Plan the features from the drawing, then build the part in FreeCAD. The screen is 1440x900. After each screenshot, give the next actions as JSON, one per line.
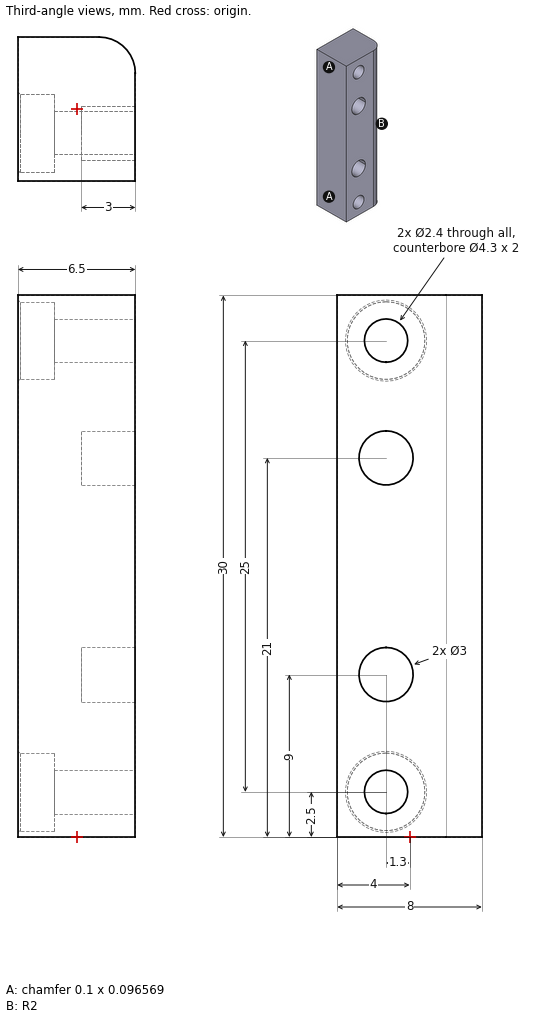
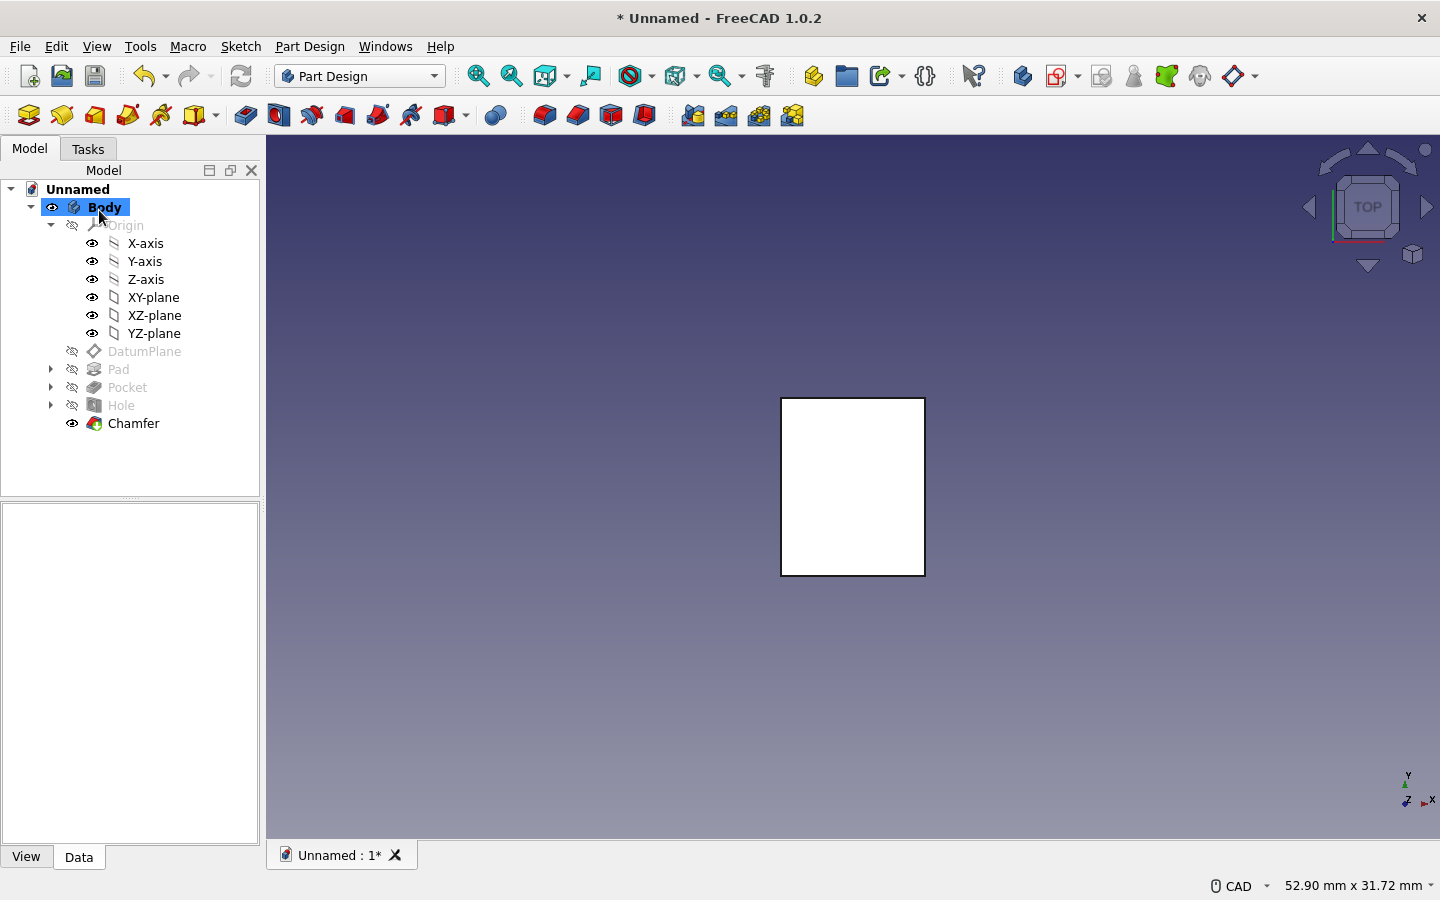
{"action": "left_click", "coordinate": [479, 76]}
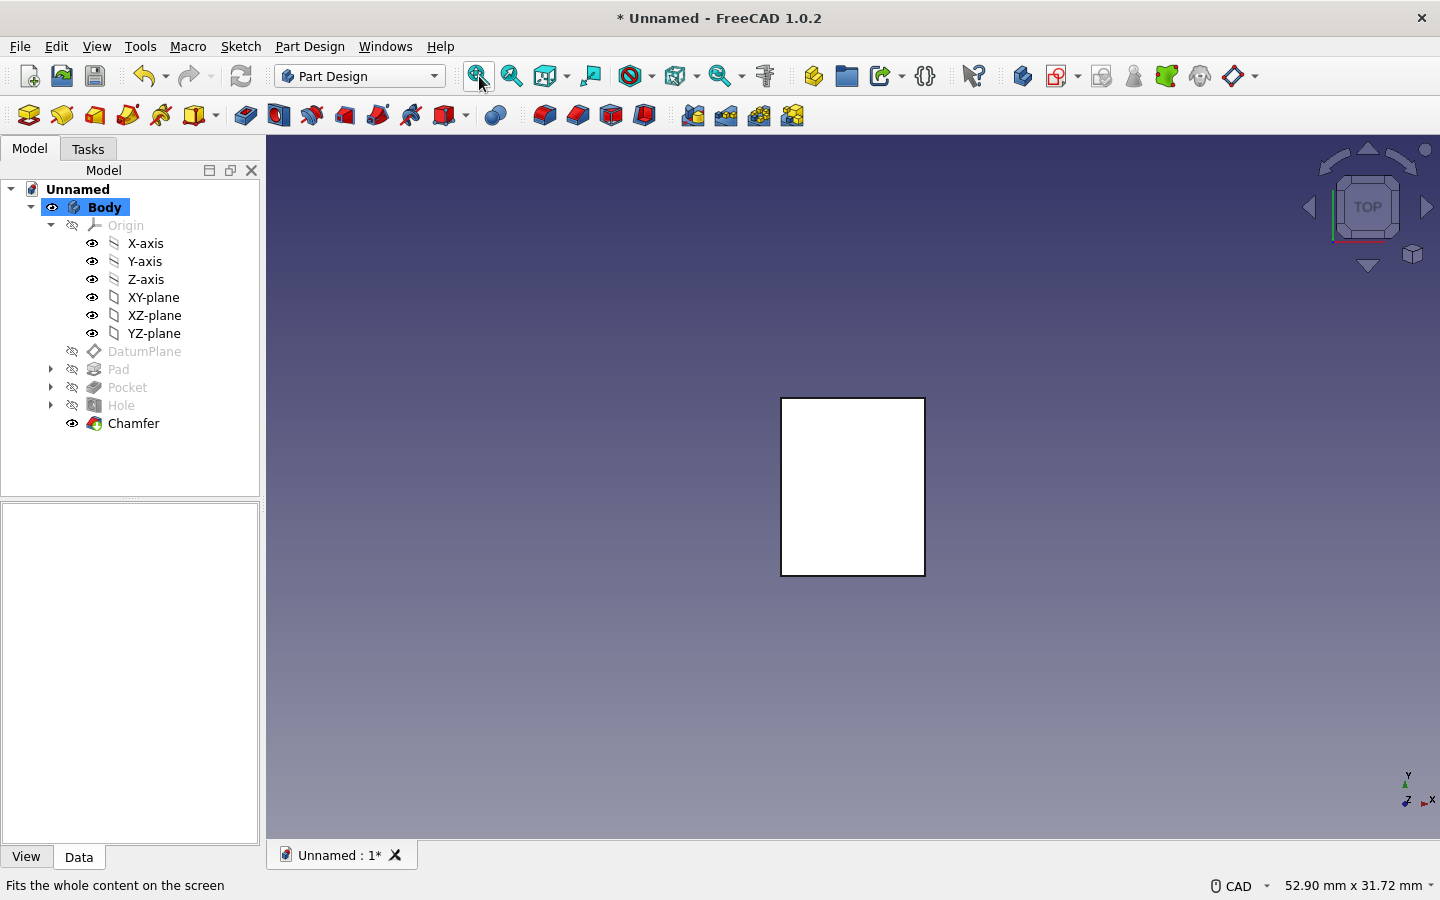
{"action": "key", "text": "1"}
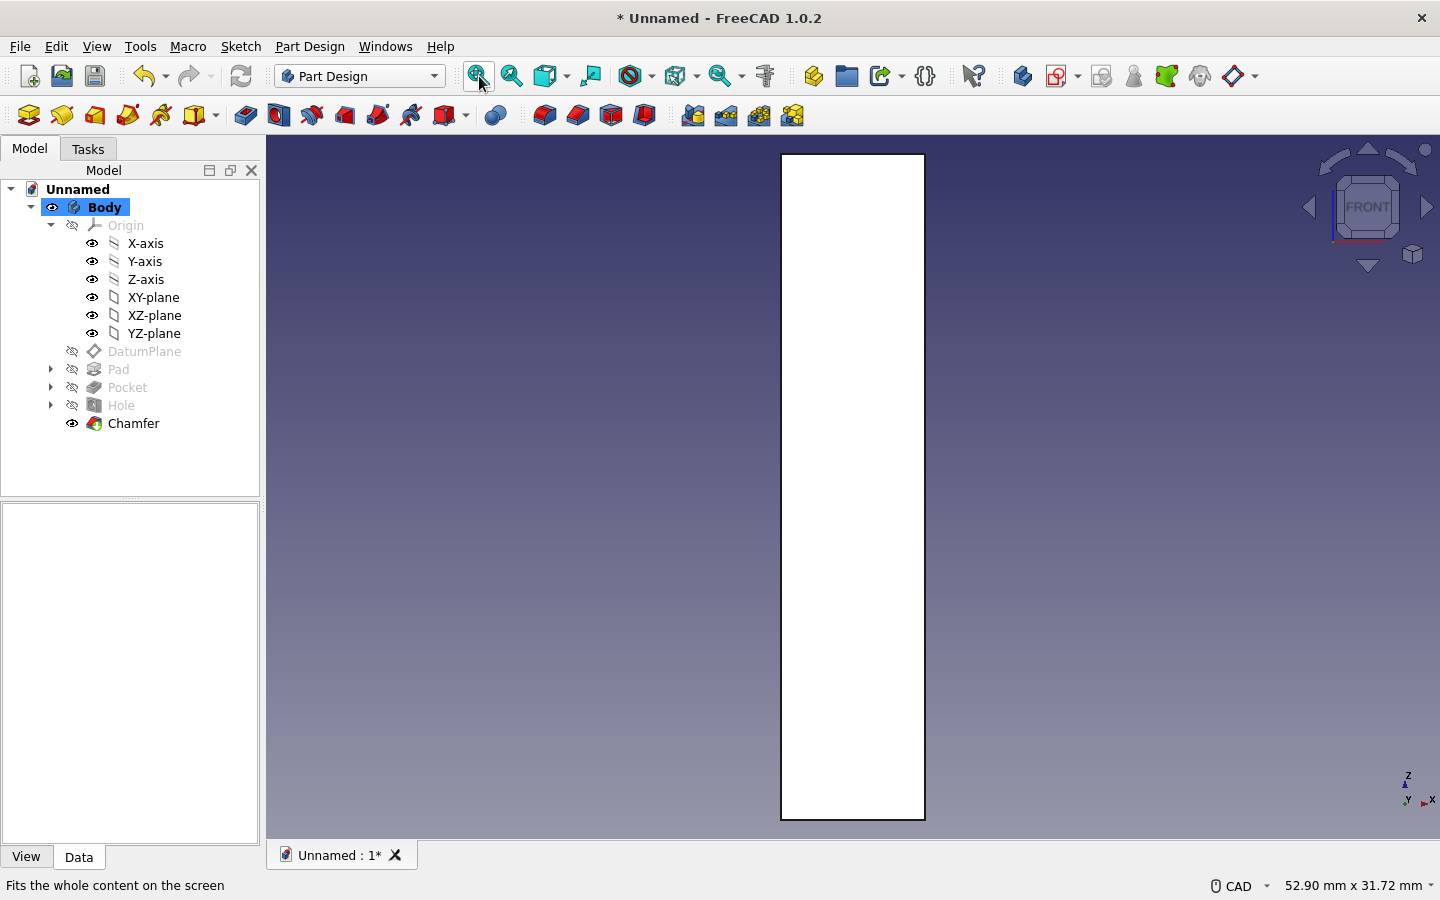
{"action": "key", "text": "3"}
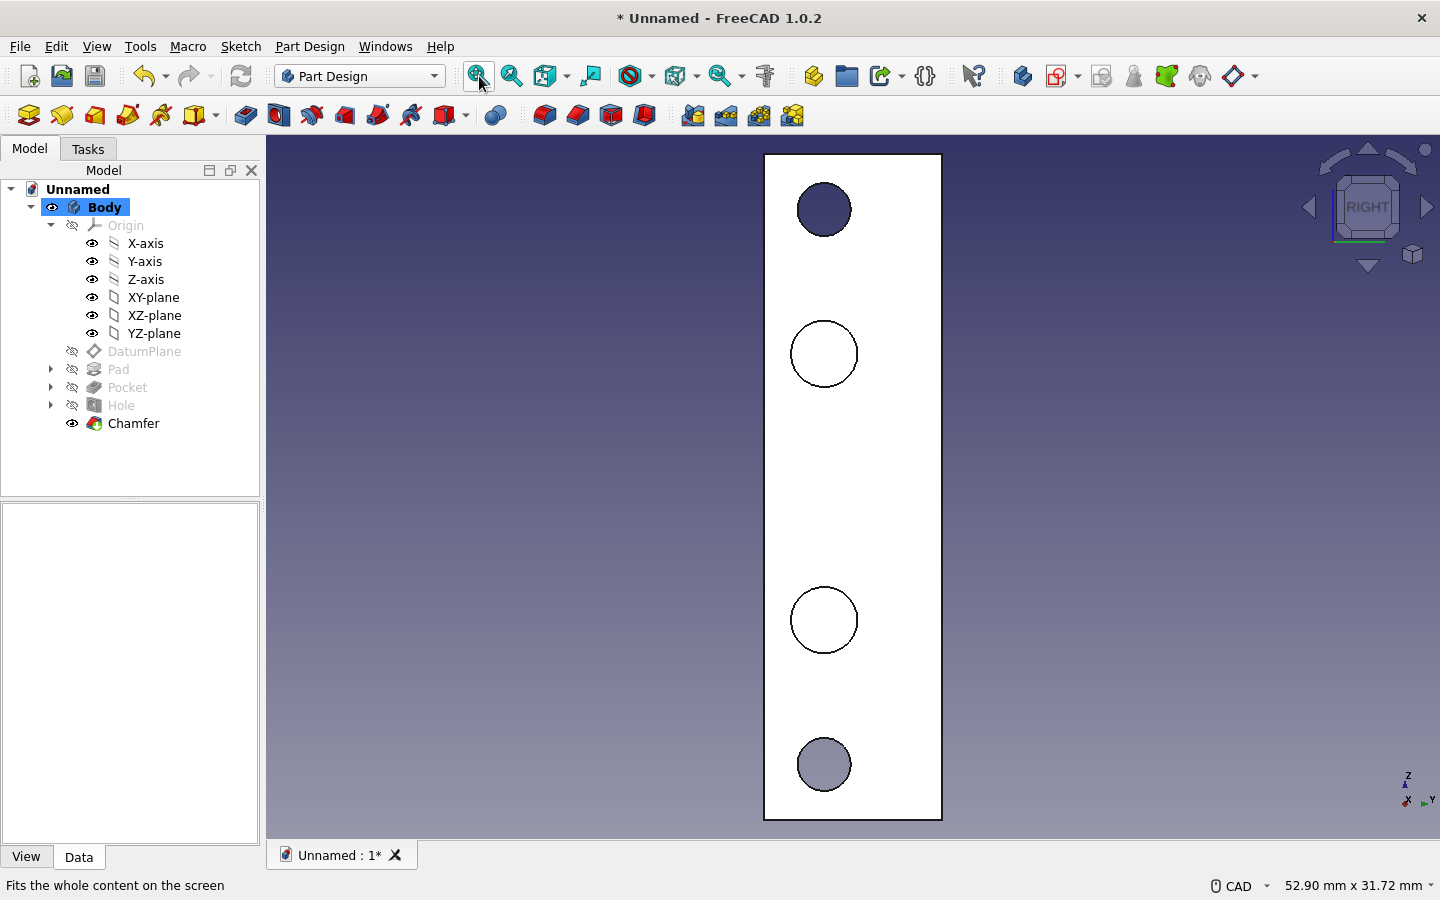
{"action": "key", "text": "5"}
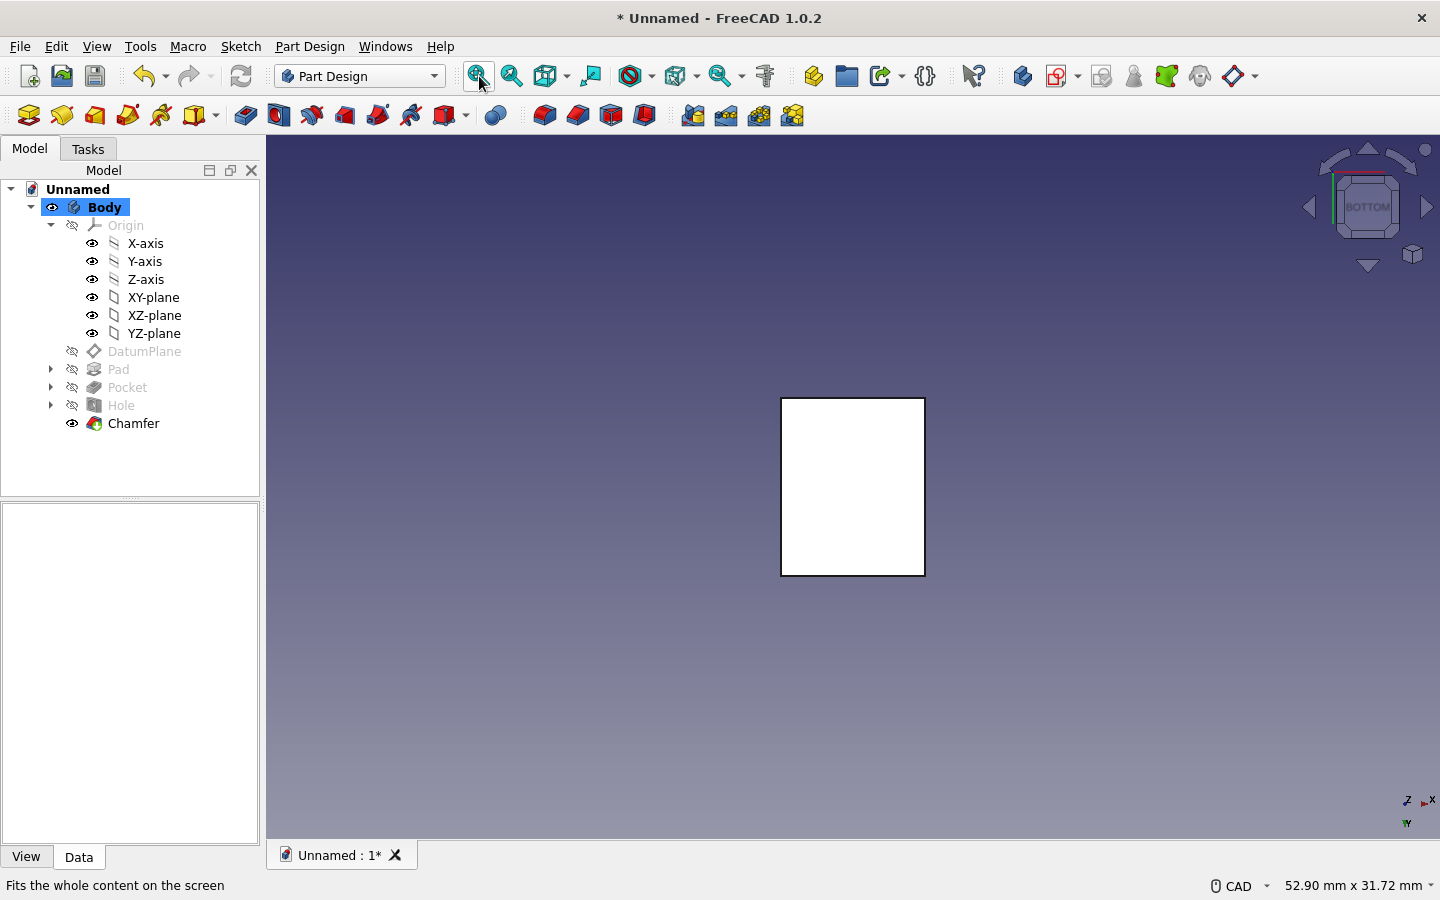
{"action": "left_click", "coordinate": [479, 76]}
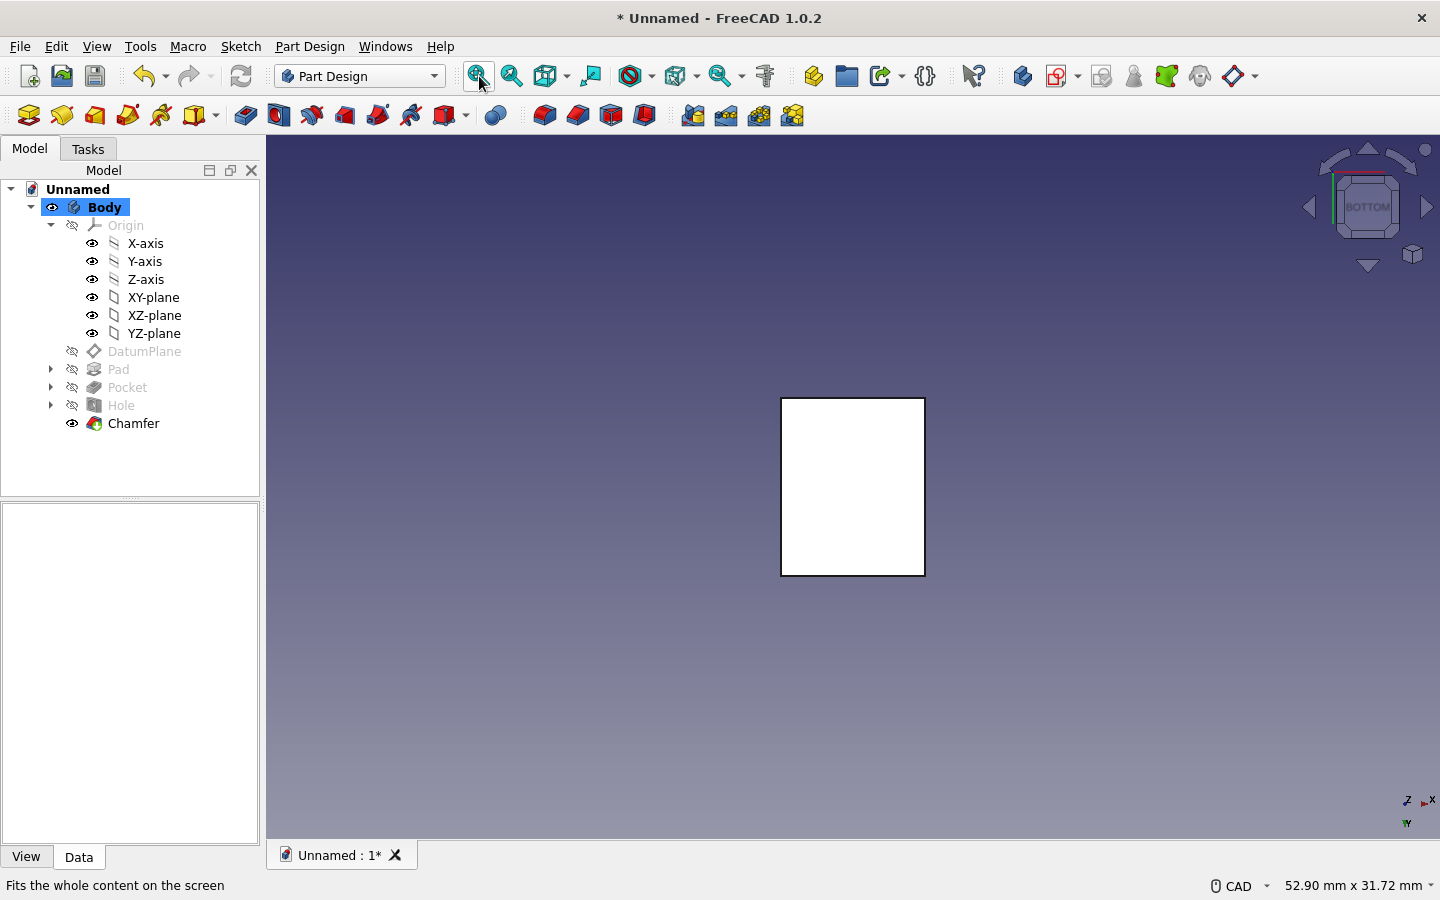
{"action": "key", "text": "4"}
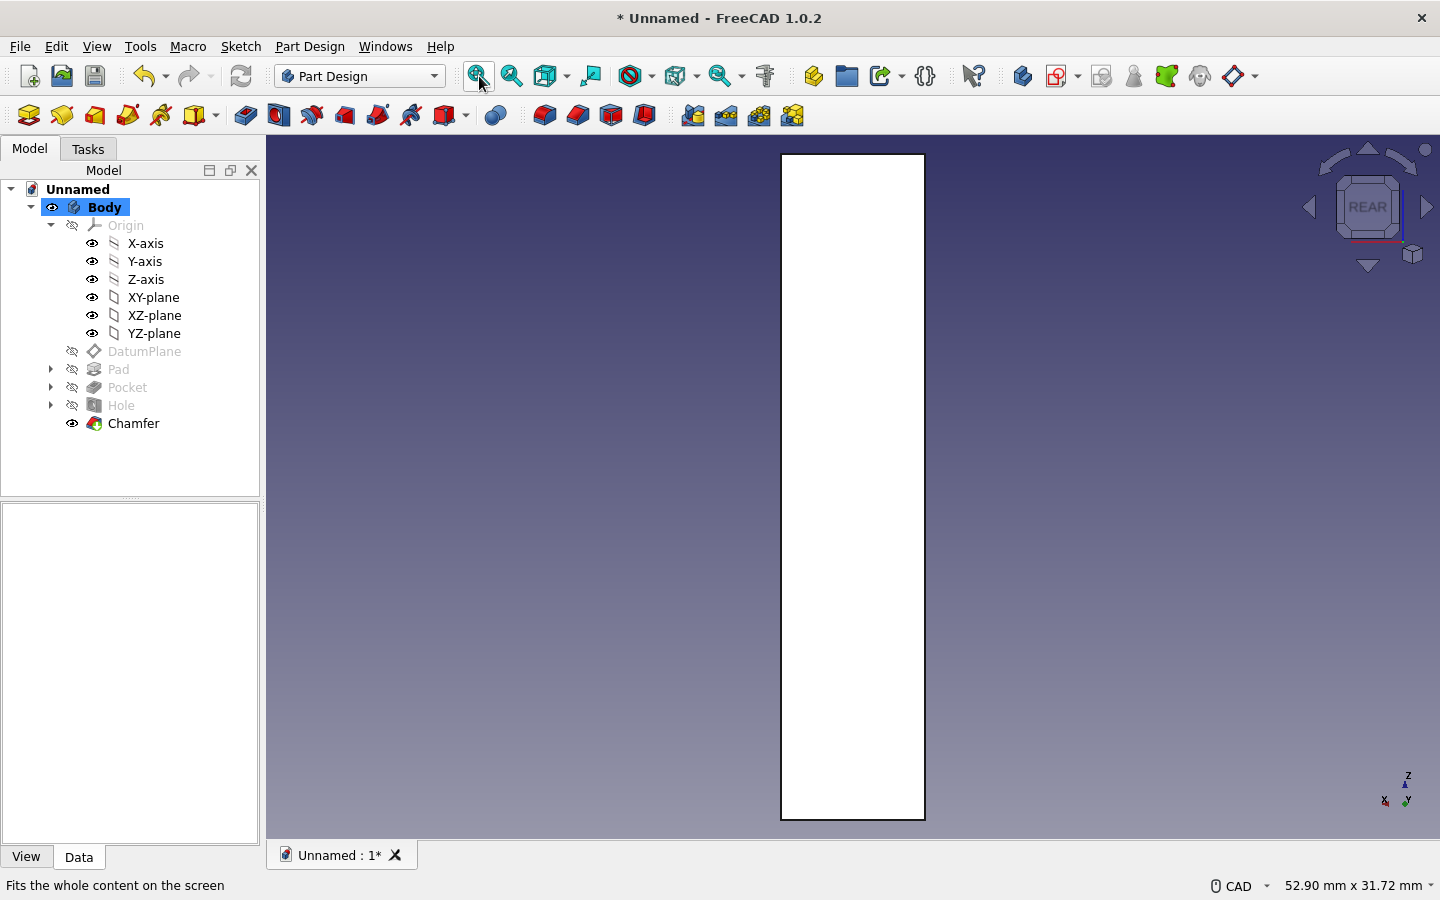
{"action": "left_click", "coordinate": [781, 486]}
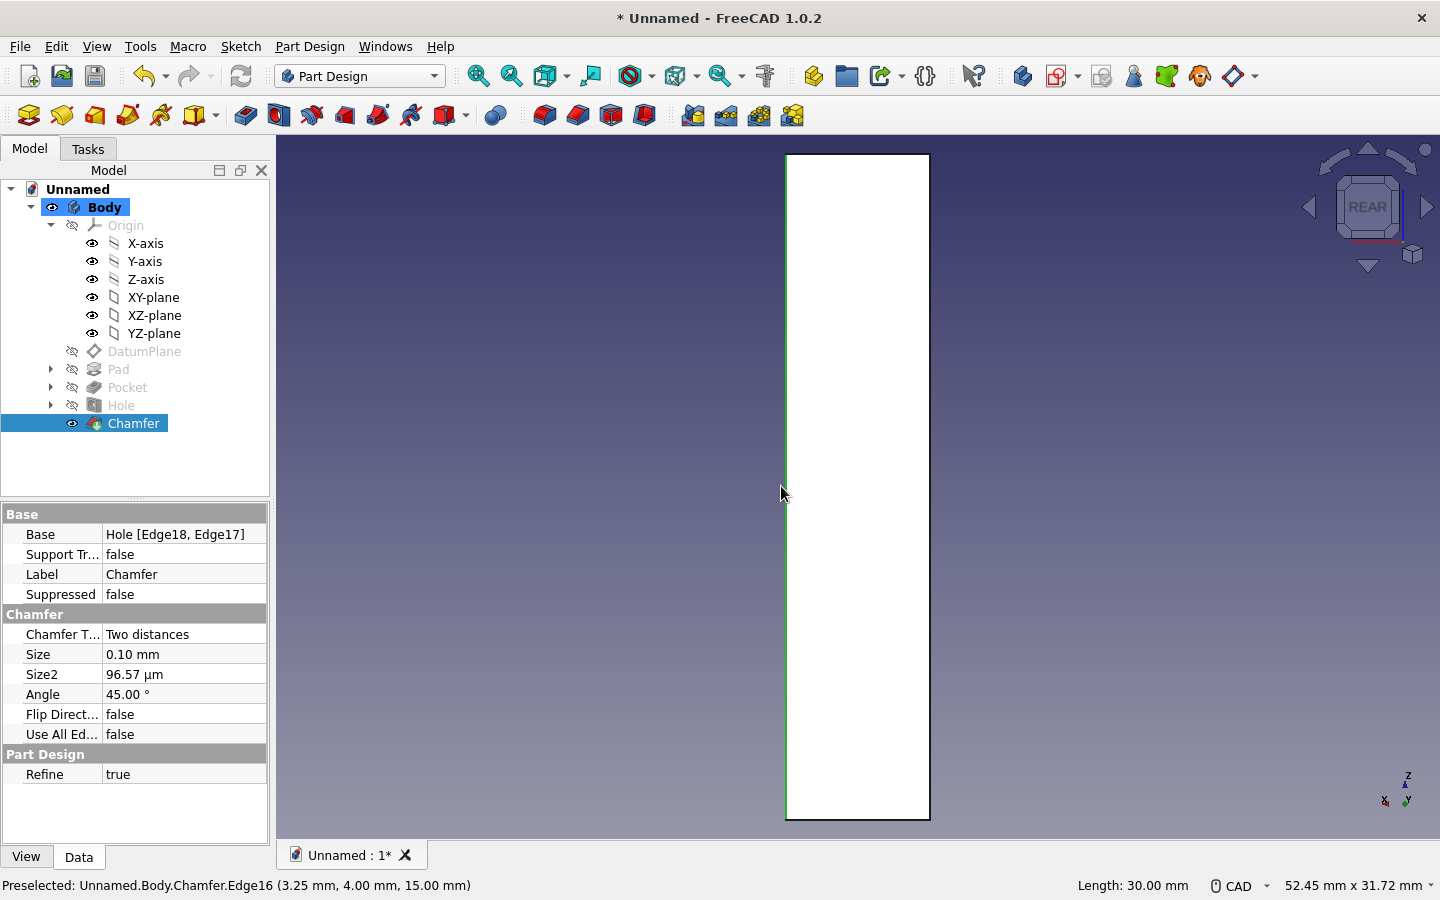
{"action": "left_click", "coordinate": [545, 116]}